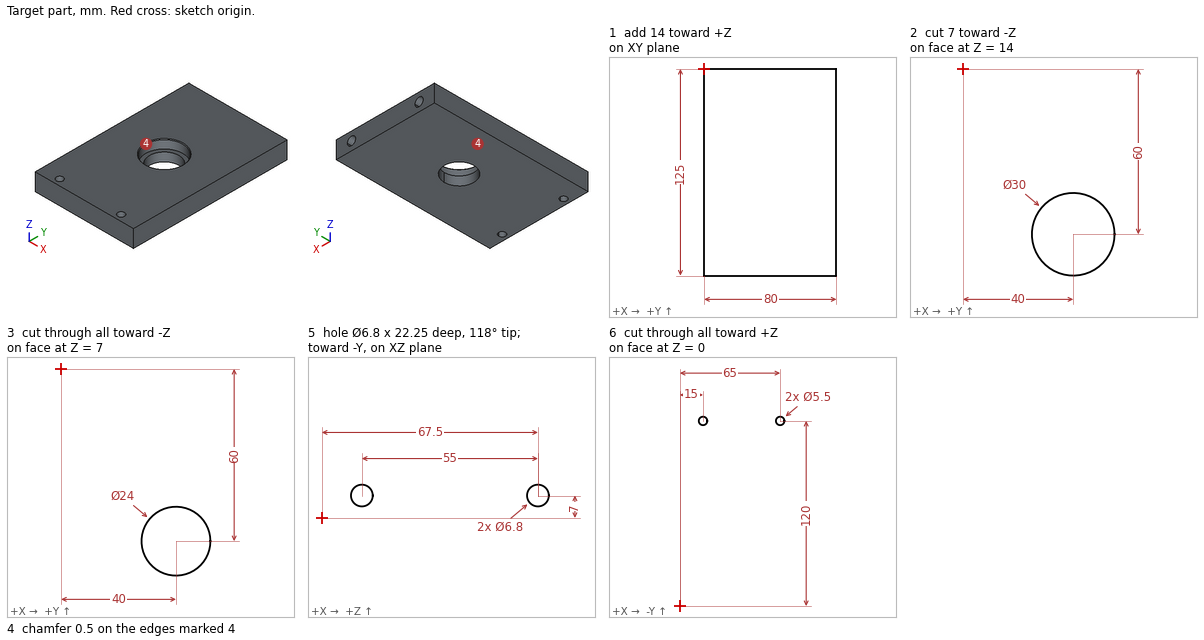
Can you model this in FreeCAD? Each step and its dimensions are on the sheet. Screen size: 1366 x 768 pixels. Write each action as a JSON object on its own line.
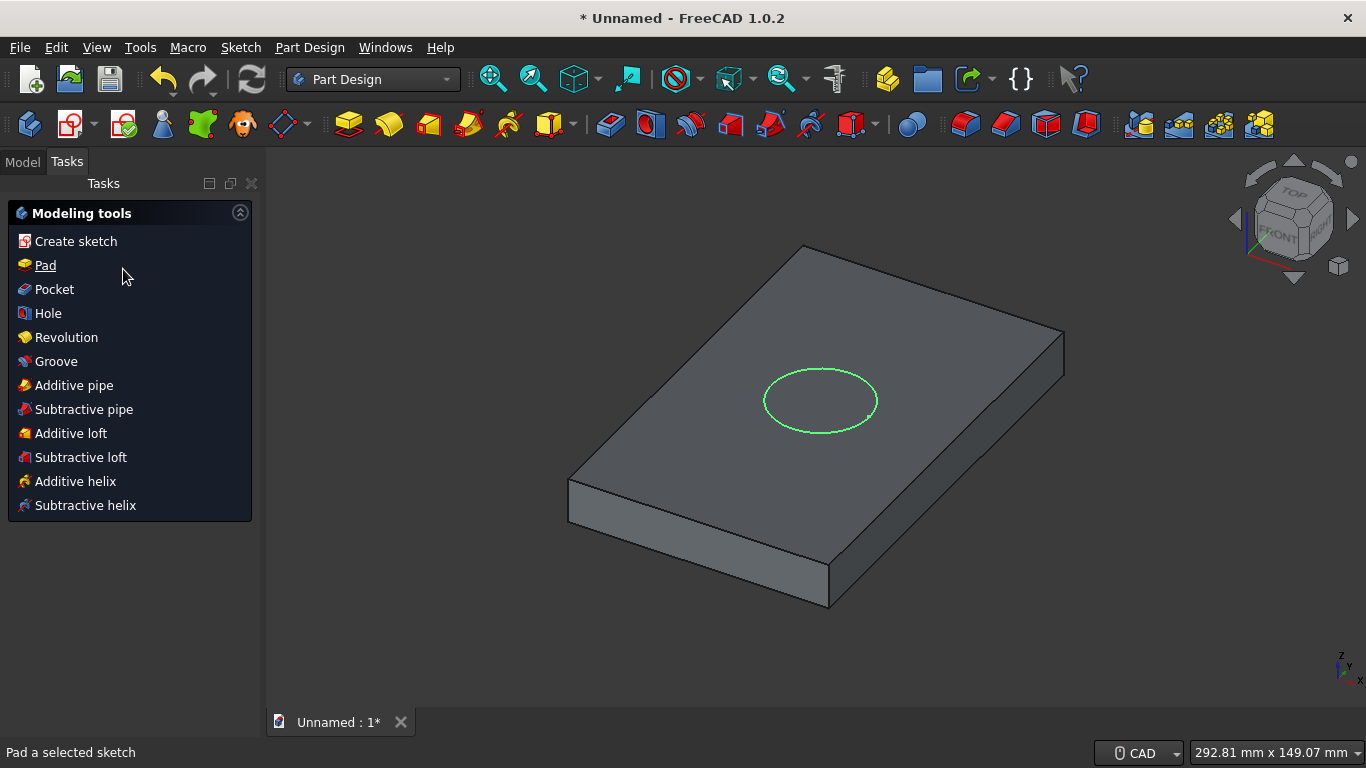
{"action": "left_click", "coordinate": [612, 124]}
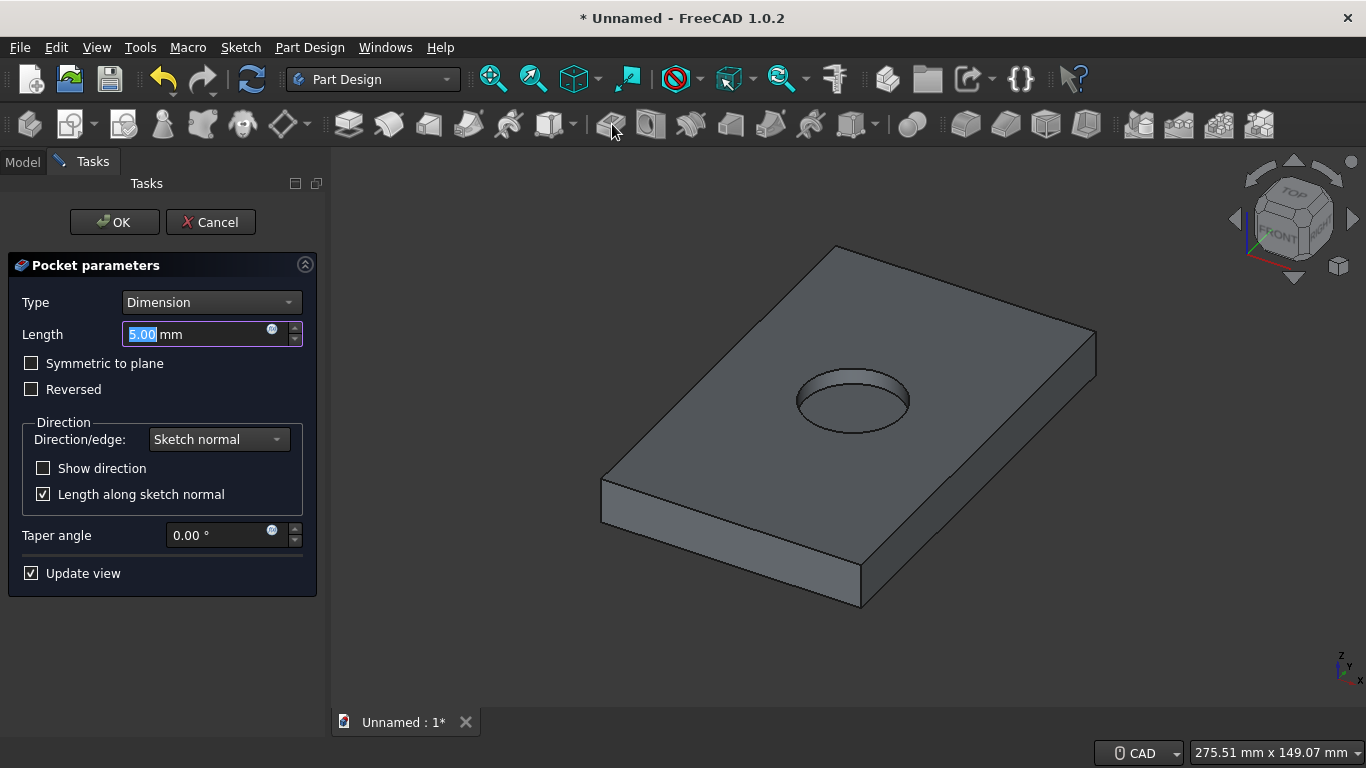
{"action": "type", "text": "7"}
{"action": "key", "text": "Tab"}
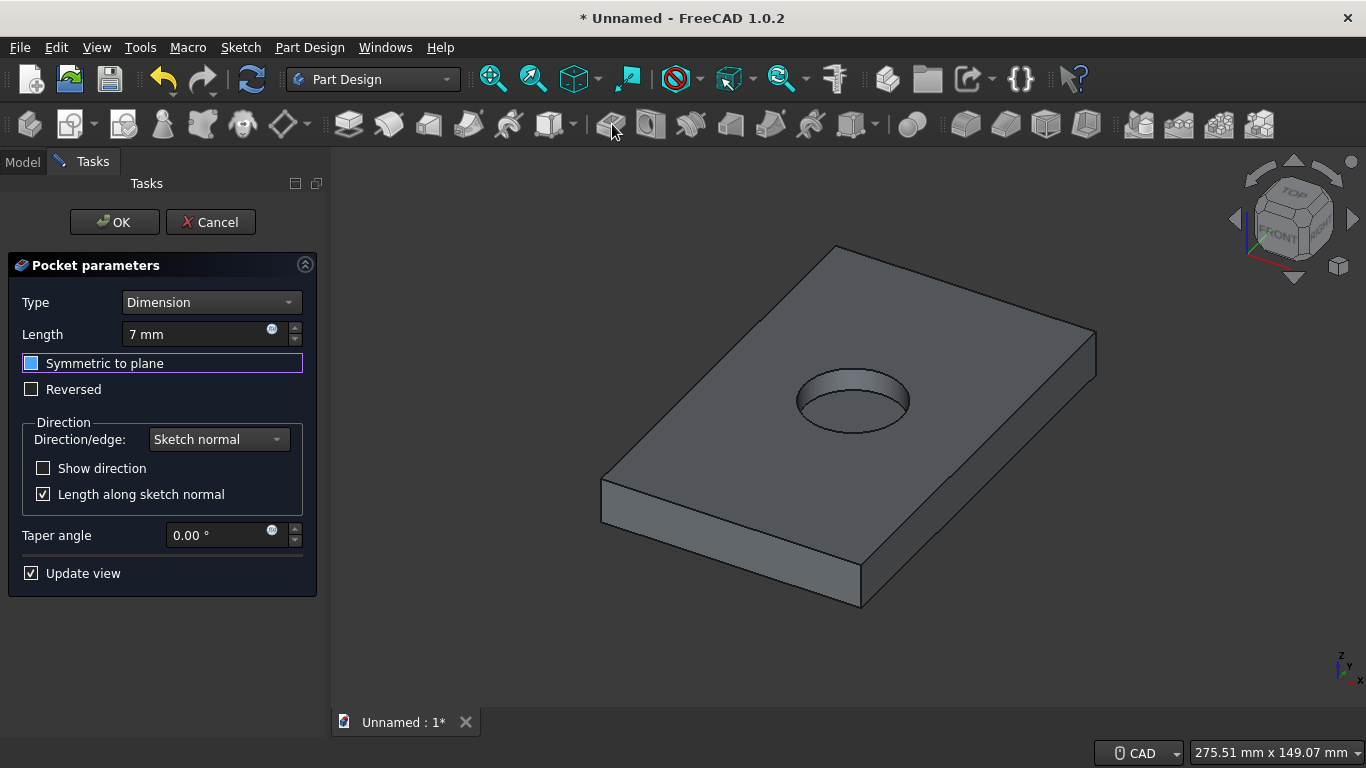
{"action": "left_click", "coordinate": [115, 222]}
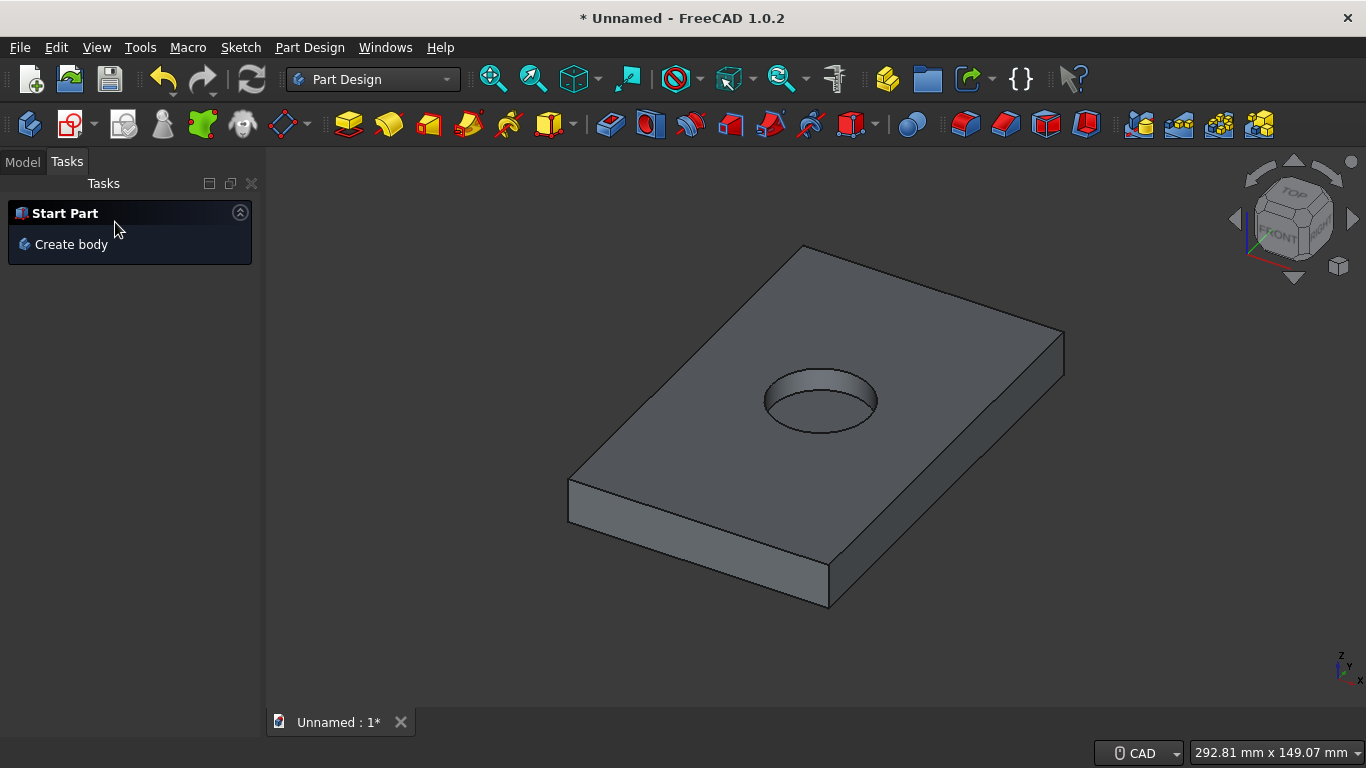
{"action": "left_click", "coordinate": [821, 421]}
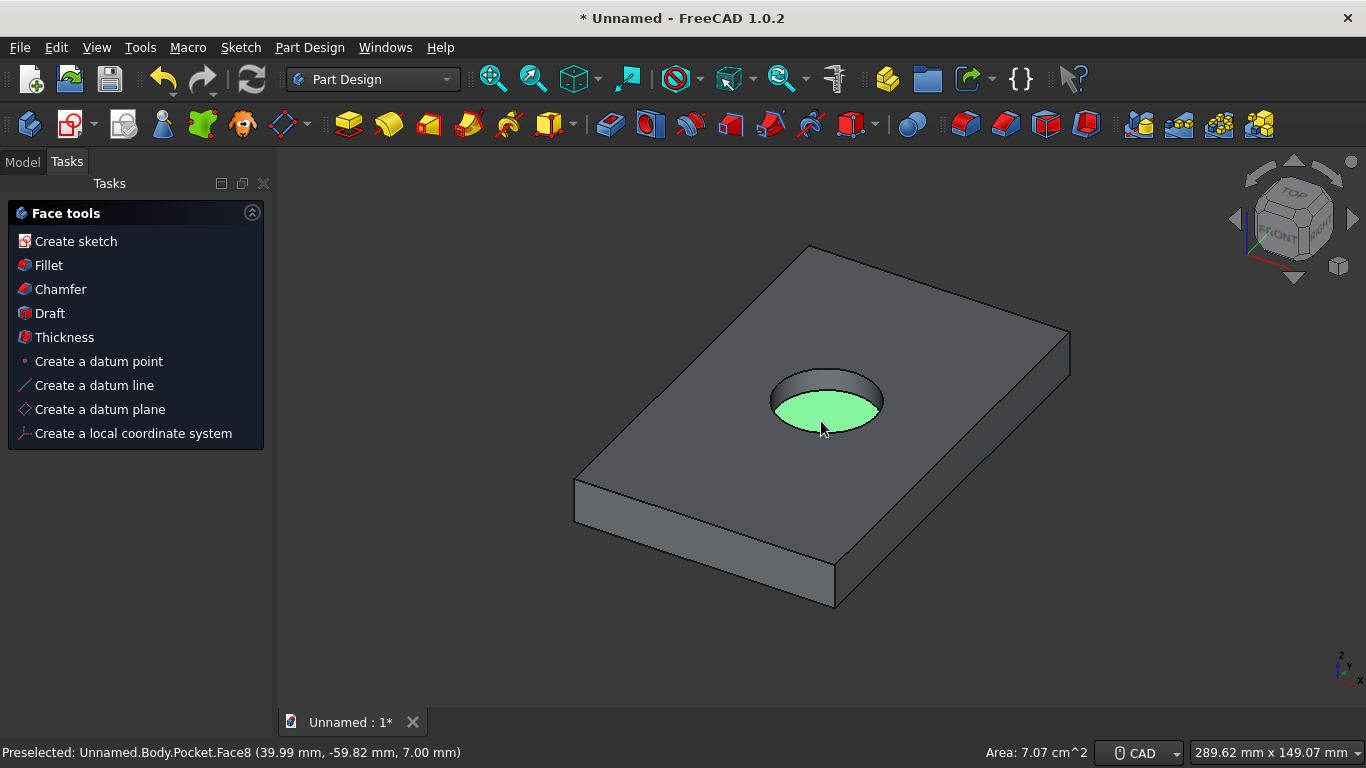
{"action": "left_click", "coordinate": [70, 124]}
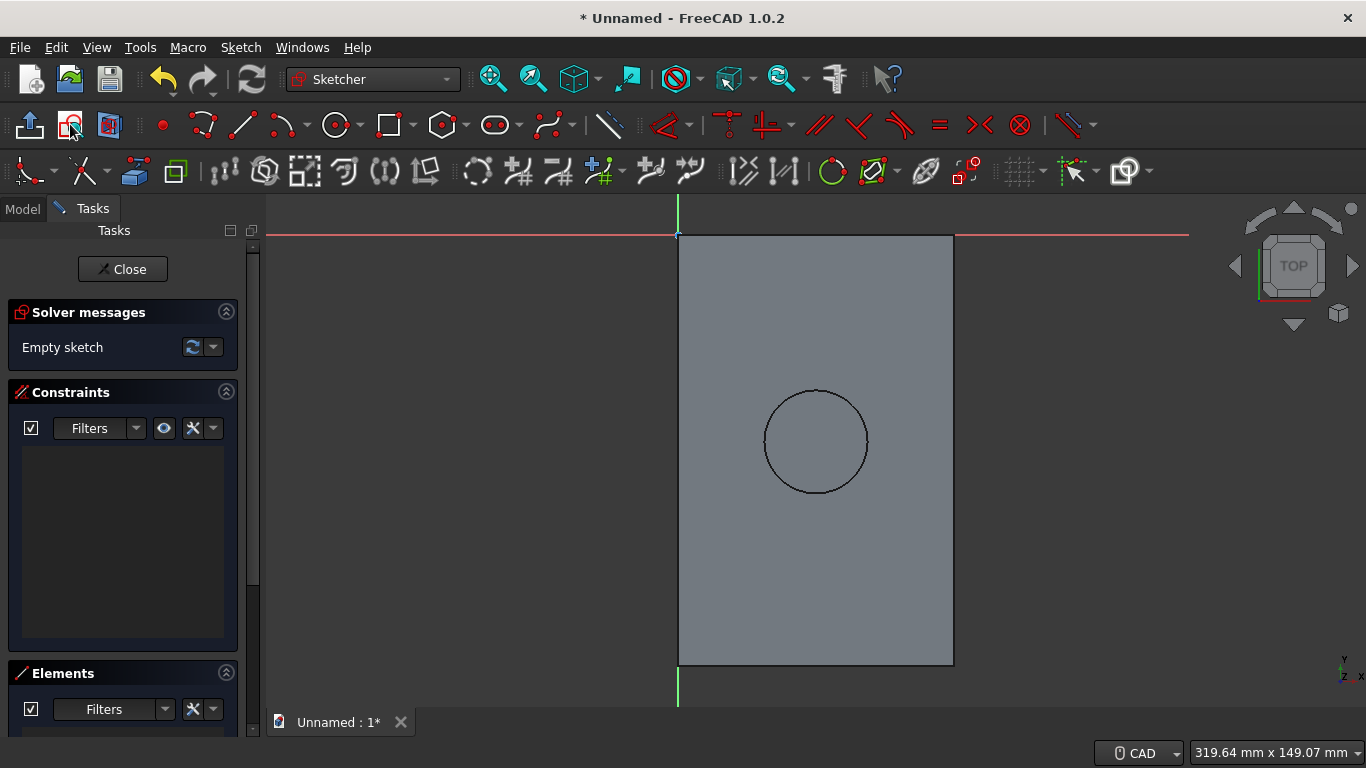
{"action": "left_click", "coordinate": [110, 126]}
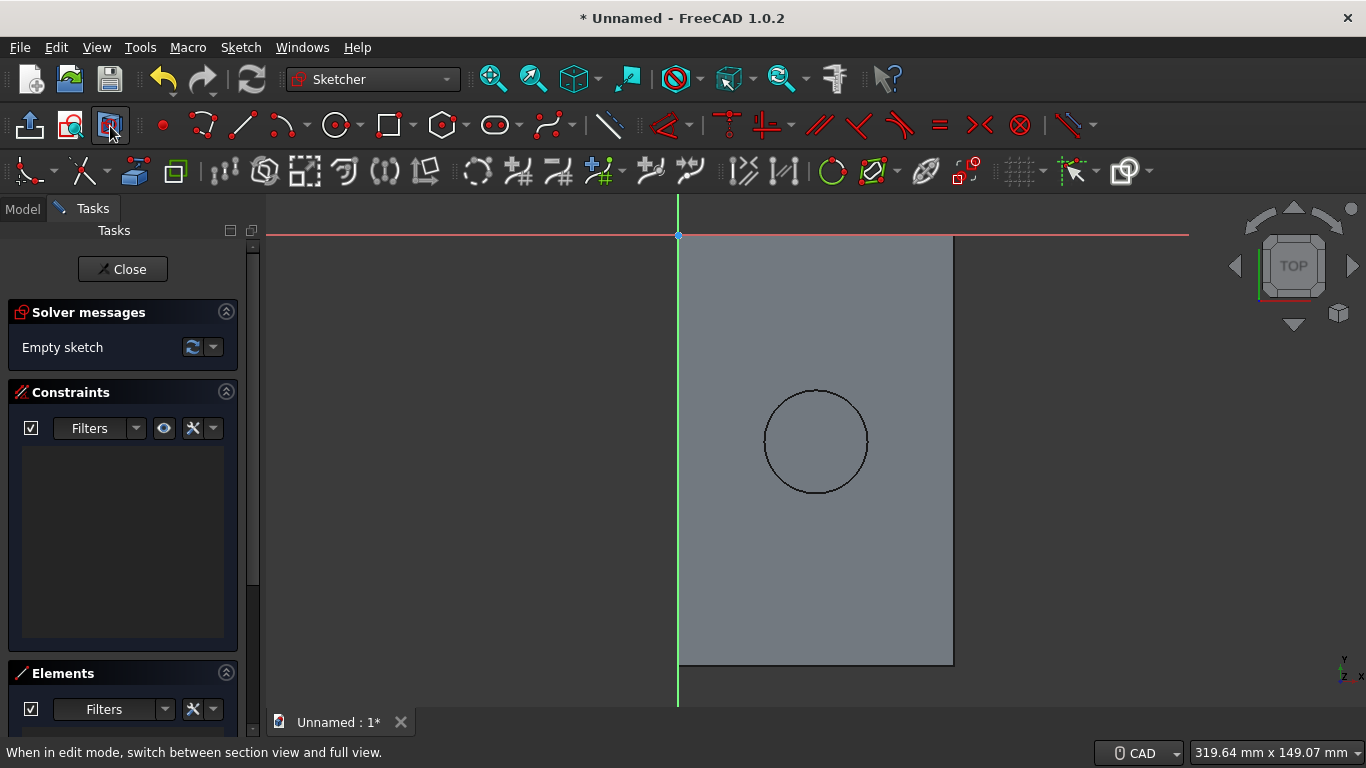
{"action": "scroll", "coordinate": [838, 439], "scroll_direction": "up", "scroll_amount": 7}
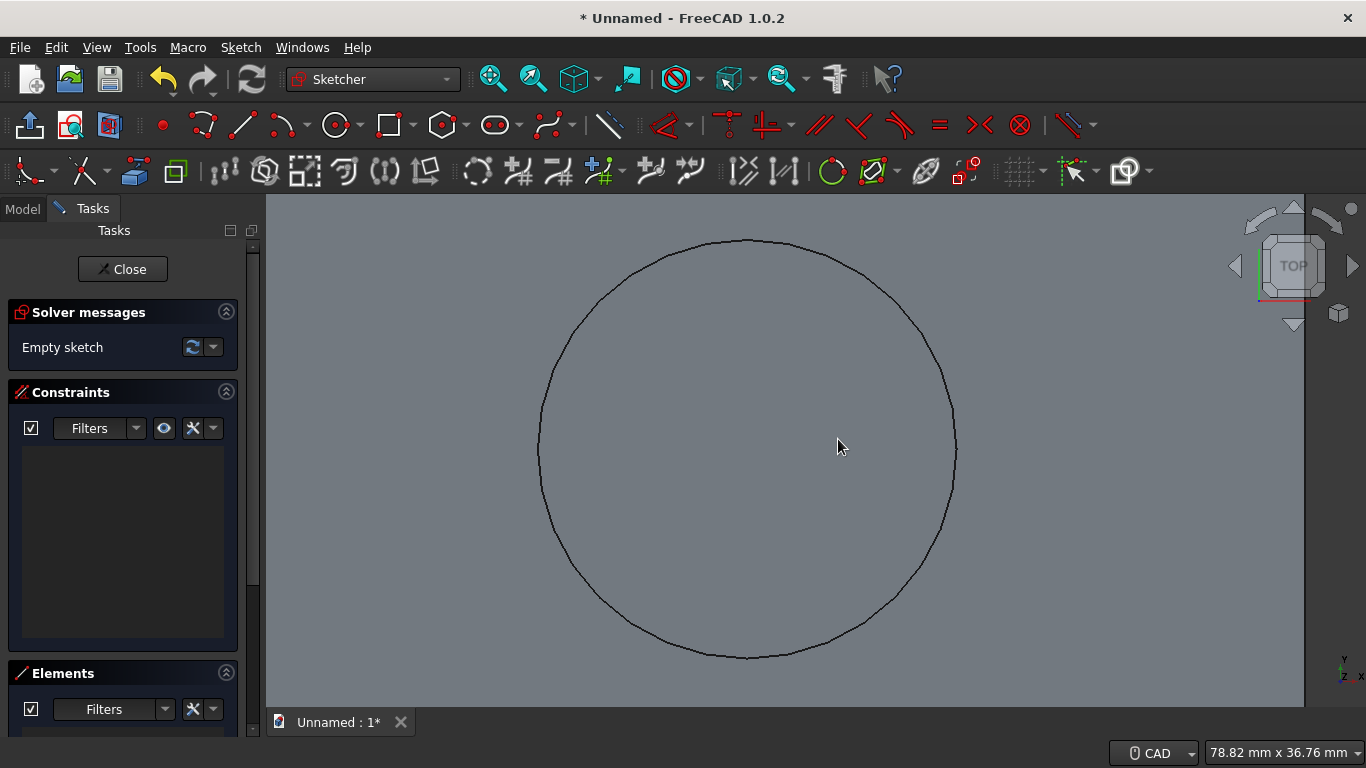
{"action": "left_click", "coordinate": [336, 126]}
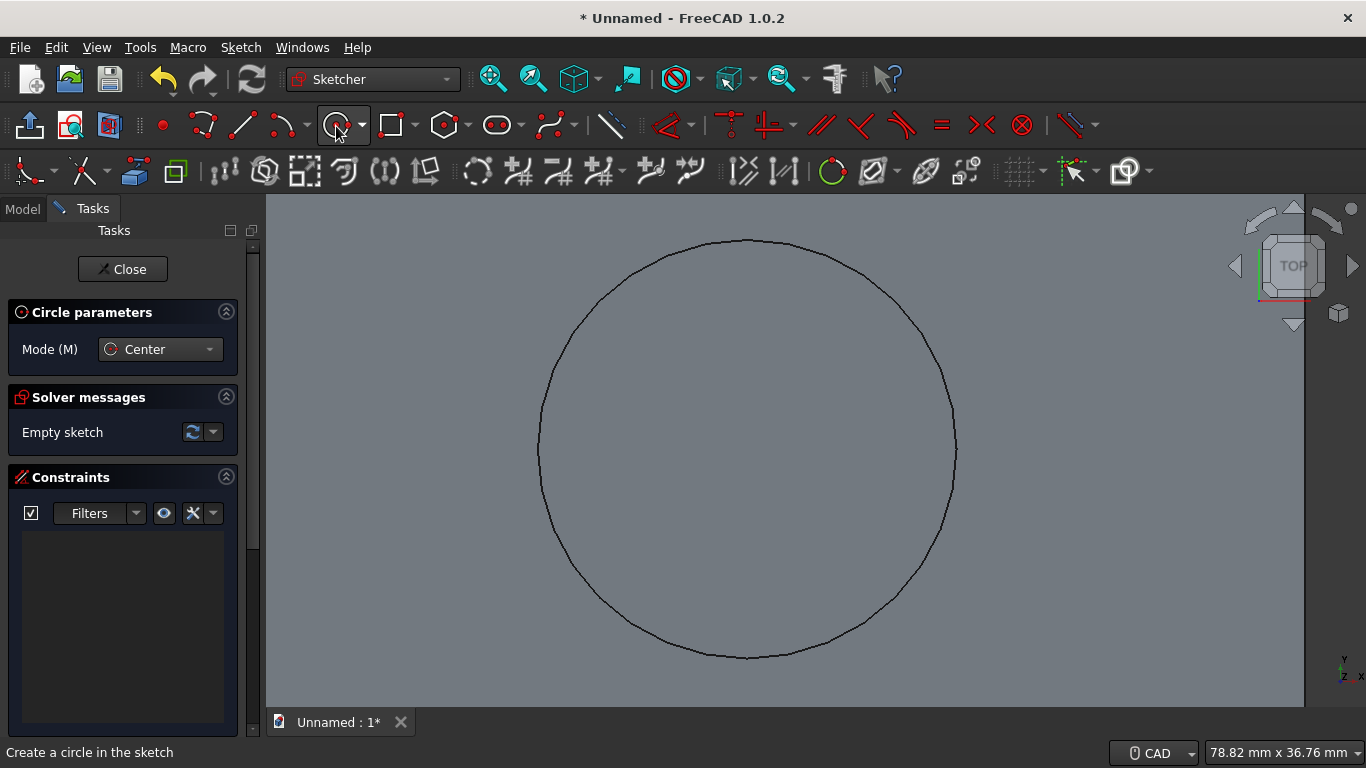
{"action": "left_click", "coordinate": [747, 449]}
{"action": "left_click", "coordinate": [866, 331]}
{"action": "key", "text": "Escape"}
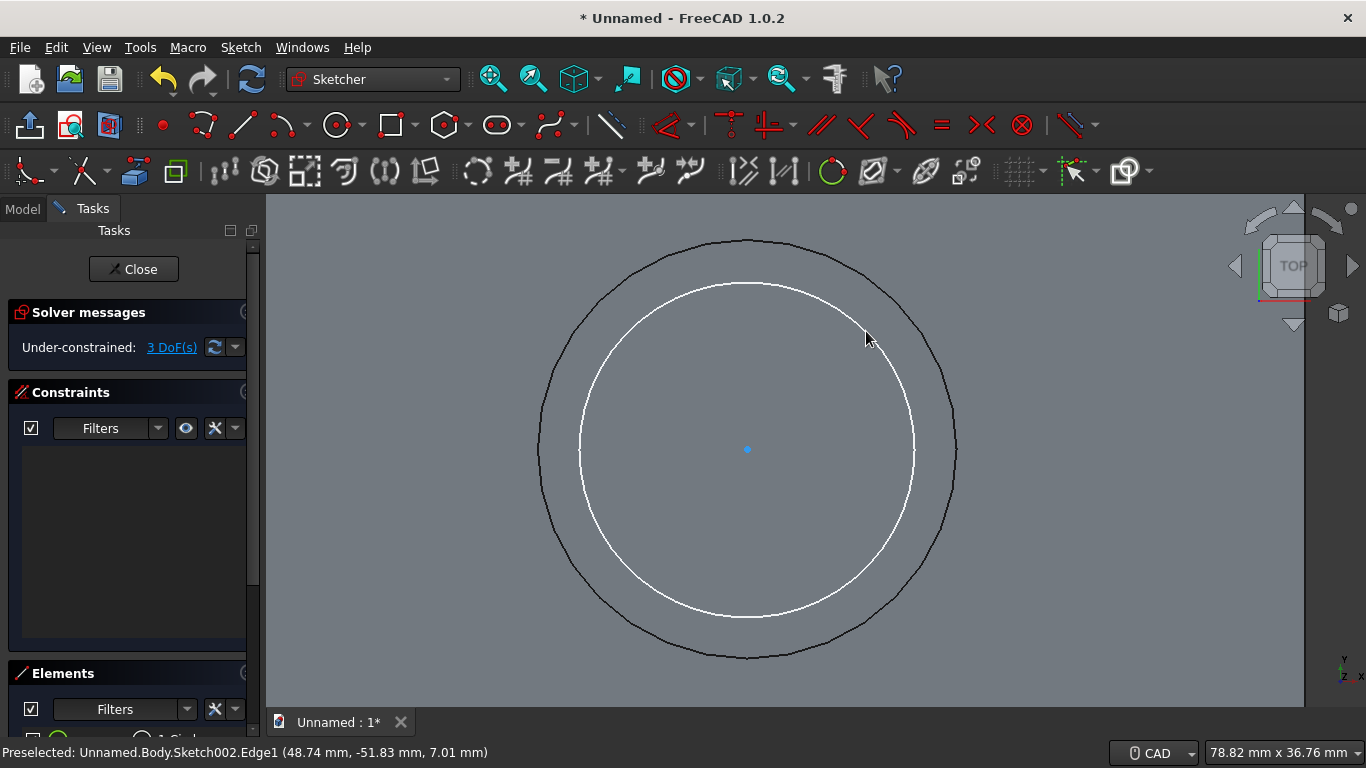
{"action": "left_click", "coordinate": [666, 126]}